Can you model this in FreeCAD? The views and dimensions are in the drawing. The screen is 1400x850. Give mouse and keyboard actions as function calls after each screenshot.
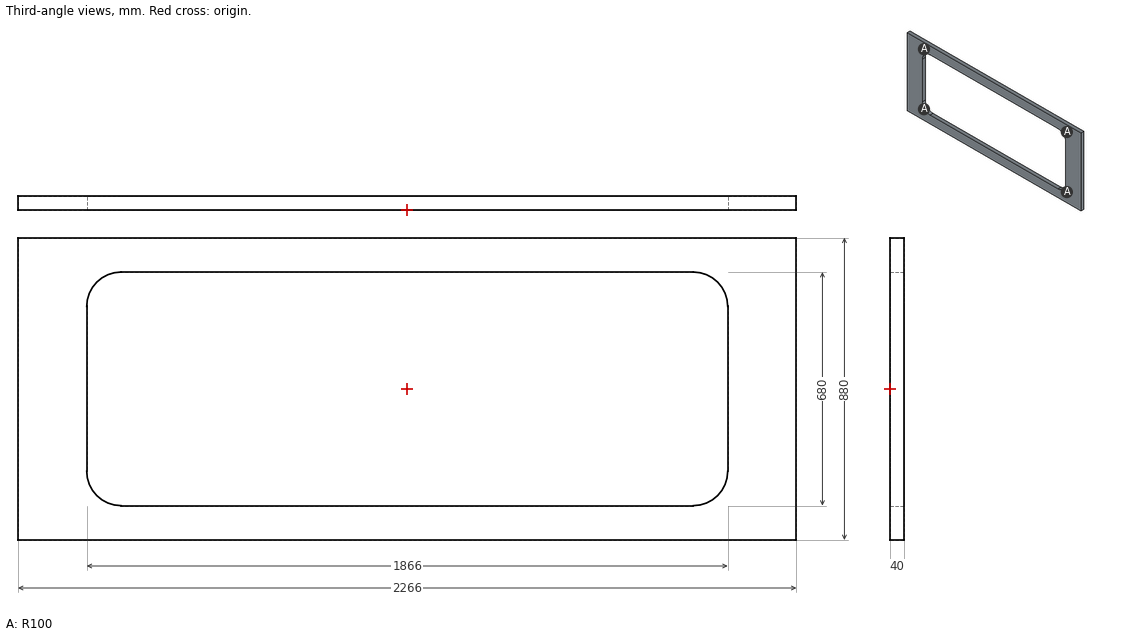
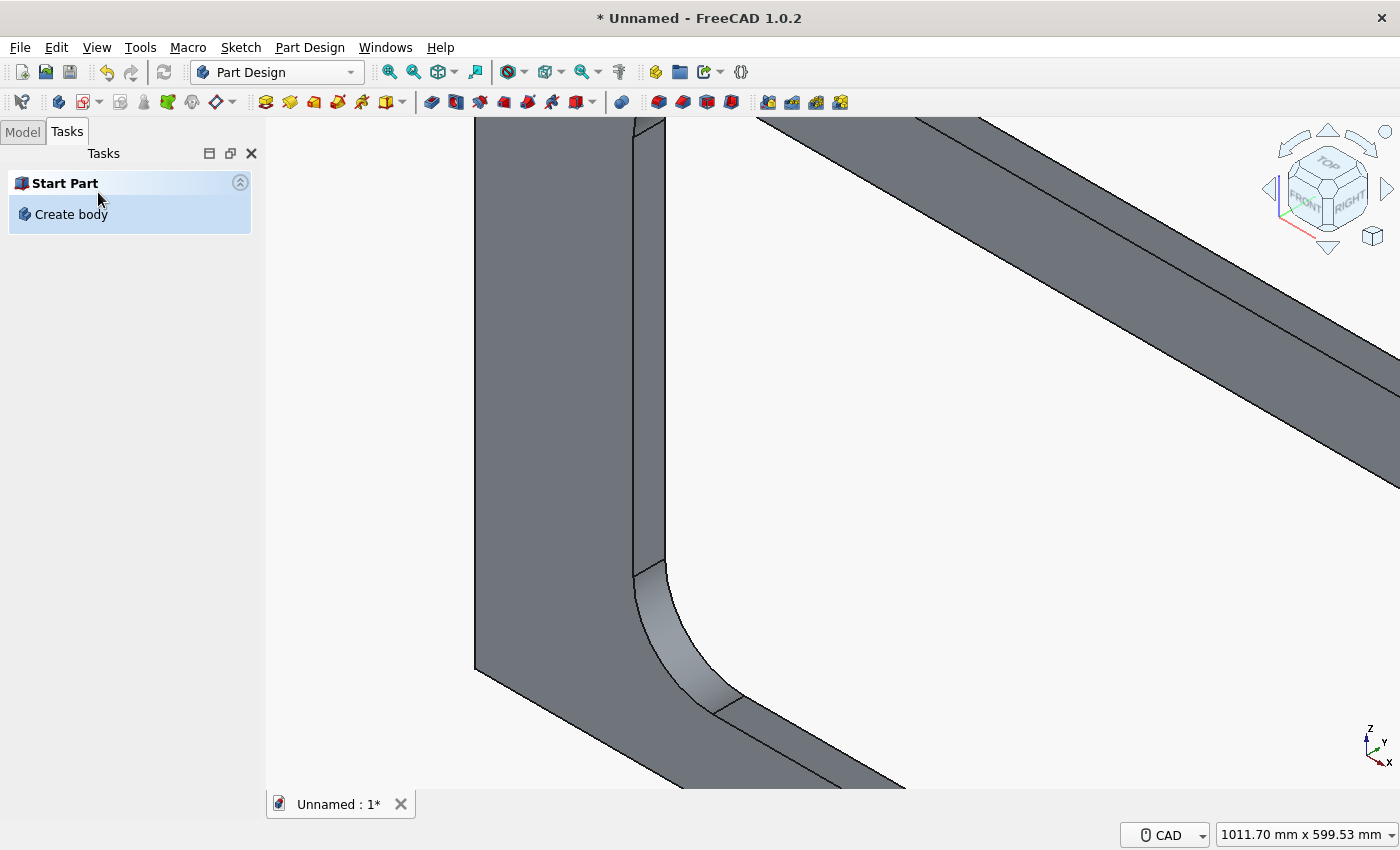
key(v)
key(f)